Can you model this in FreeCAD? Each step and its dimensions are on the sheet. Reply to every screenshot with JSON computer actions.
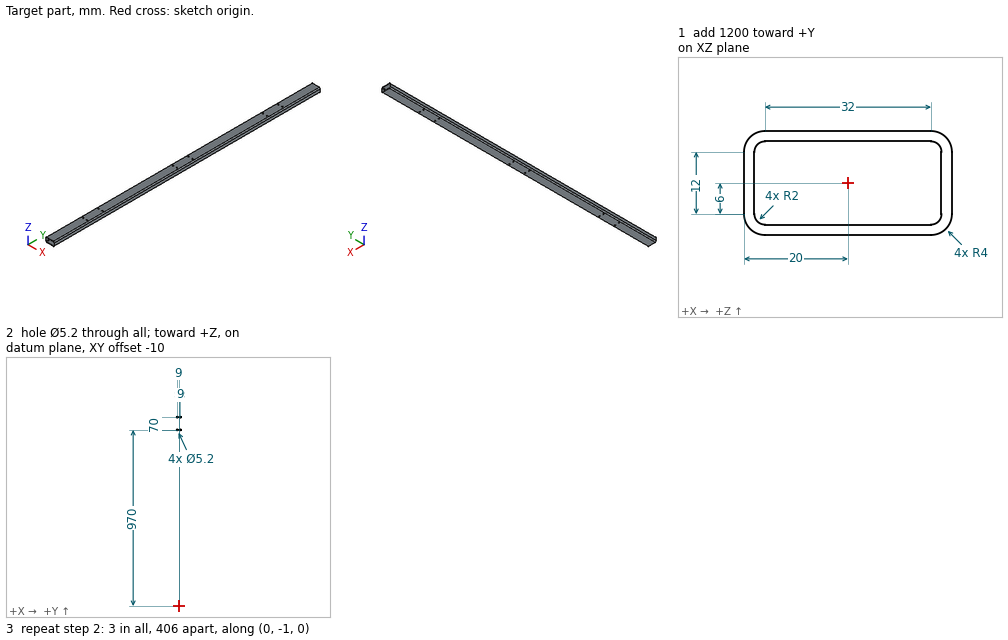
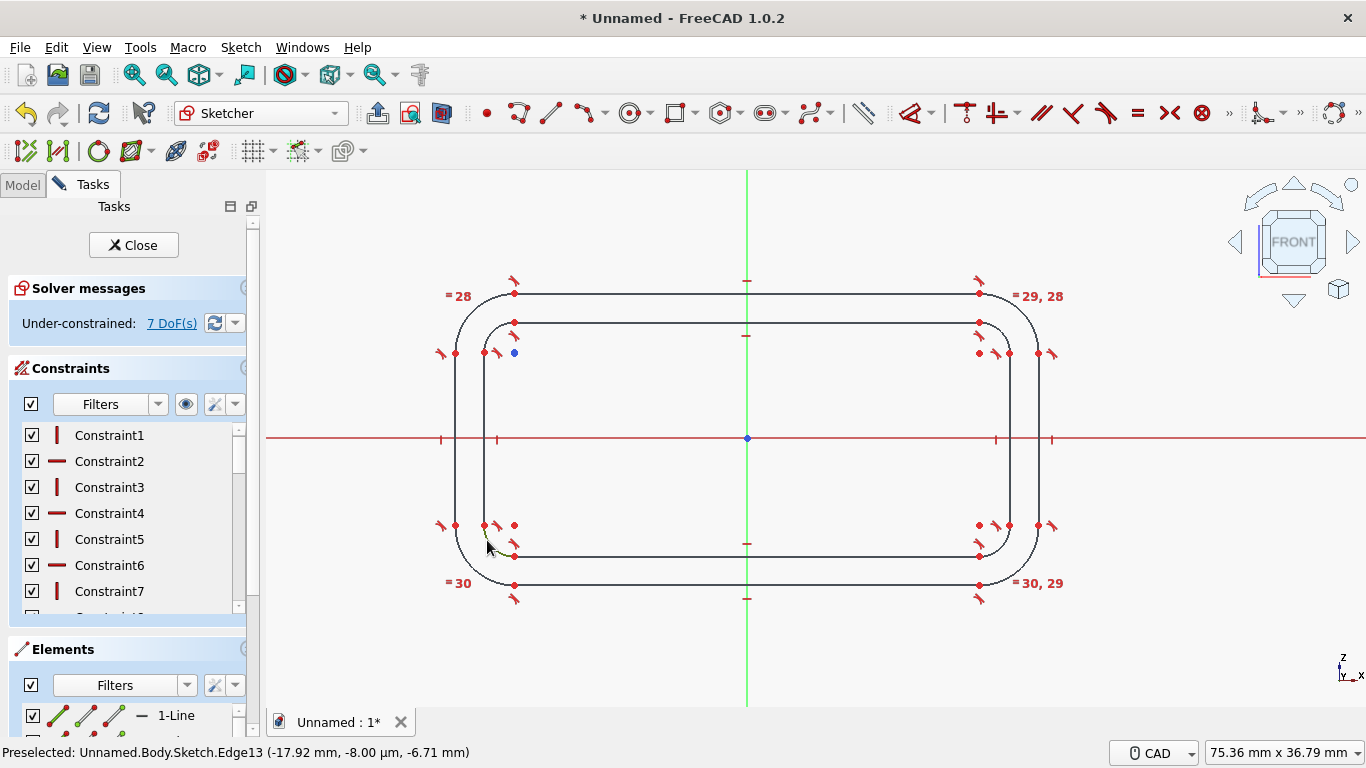
{"action": "left_click", "coordinate": [501, 326]}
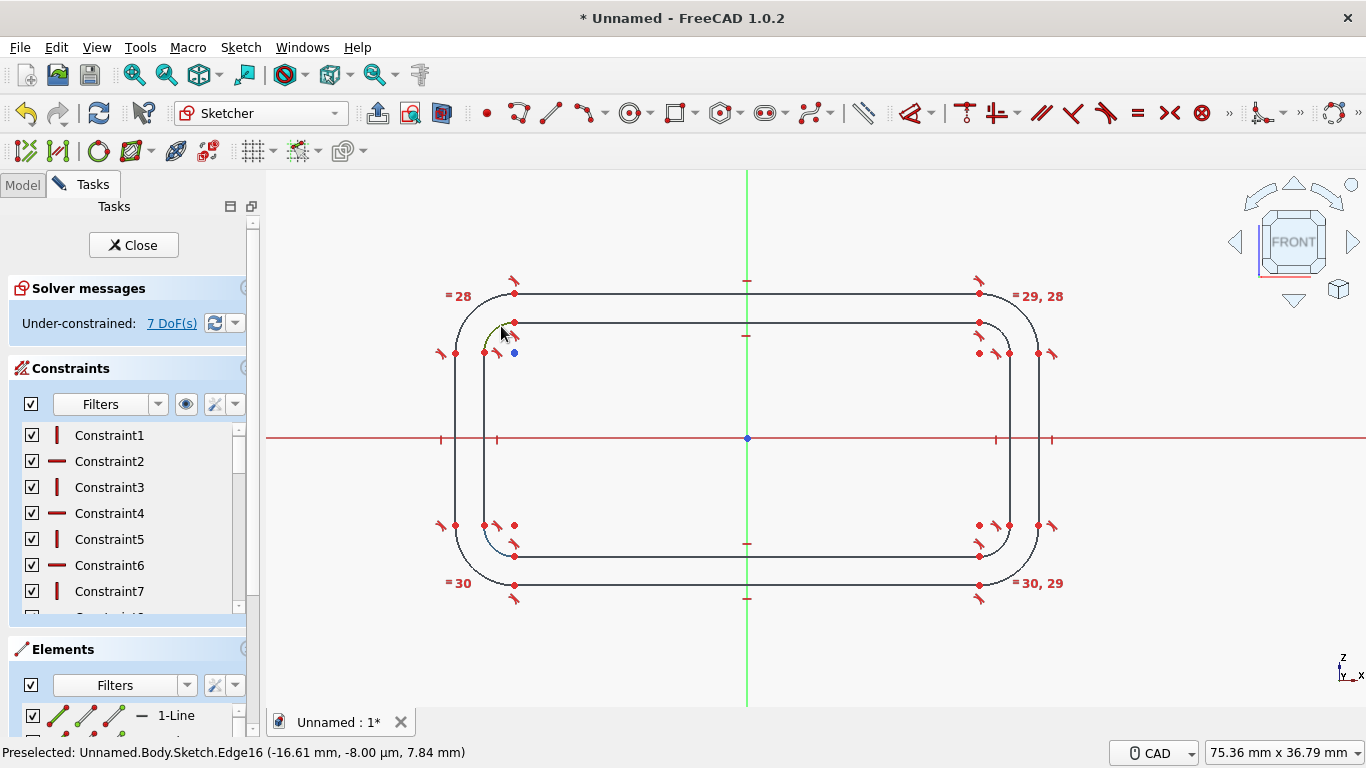
{"action": "left_click", "coordinate": [1138, 114]}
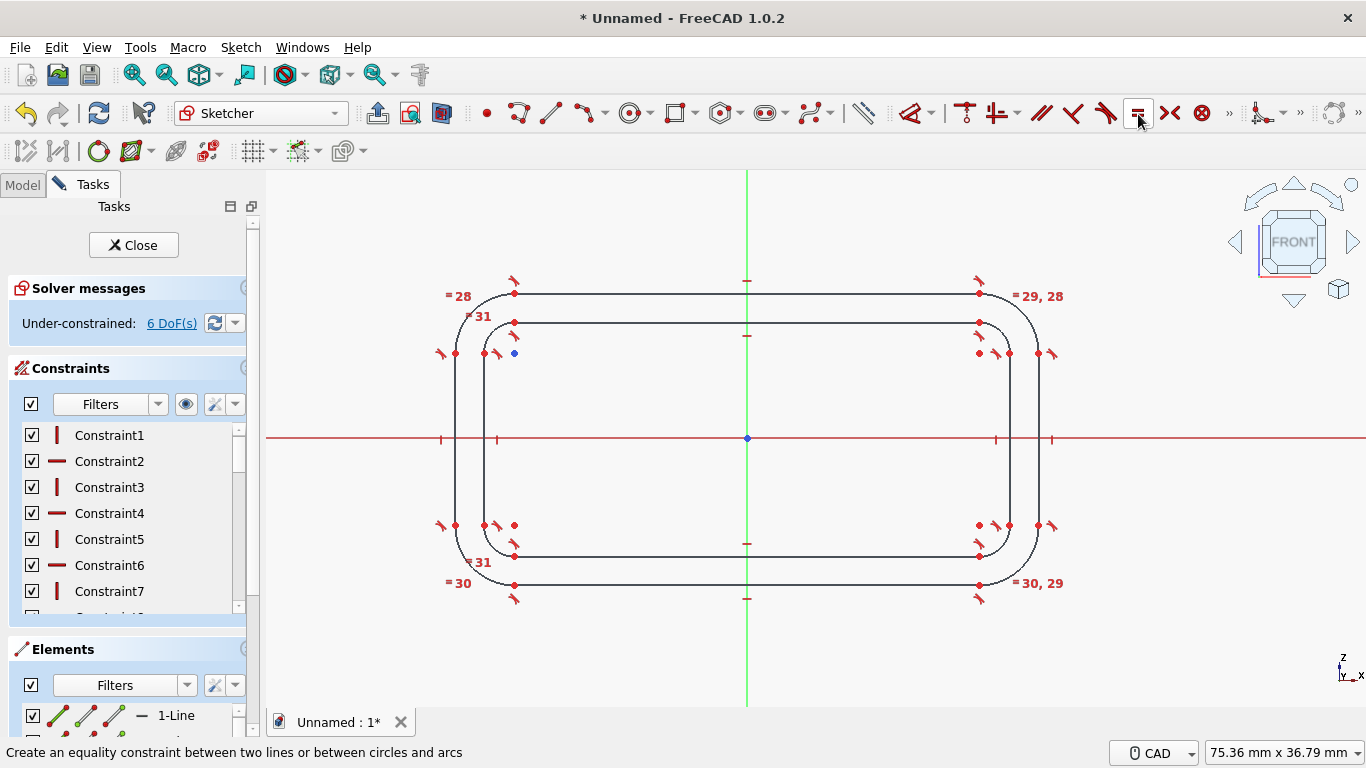
{"action": "left_click", "coordinate": [910, 114]}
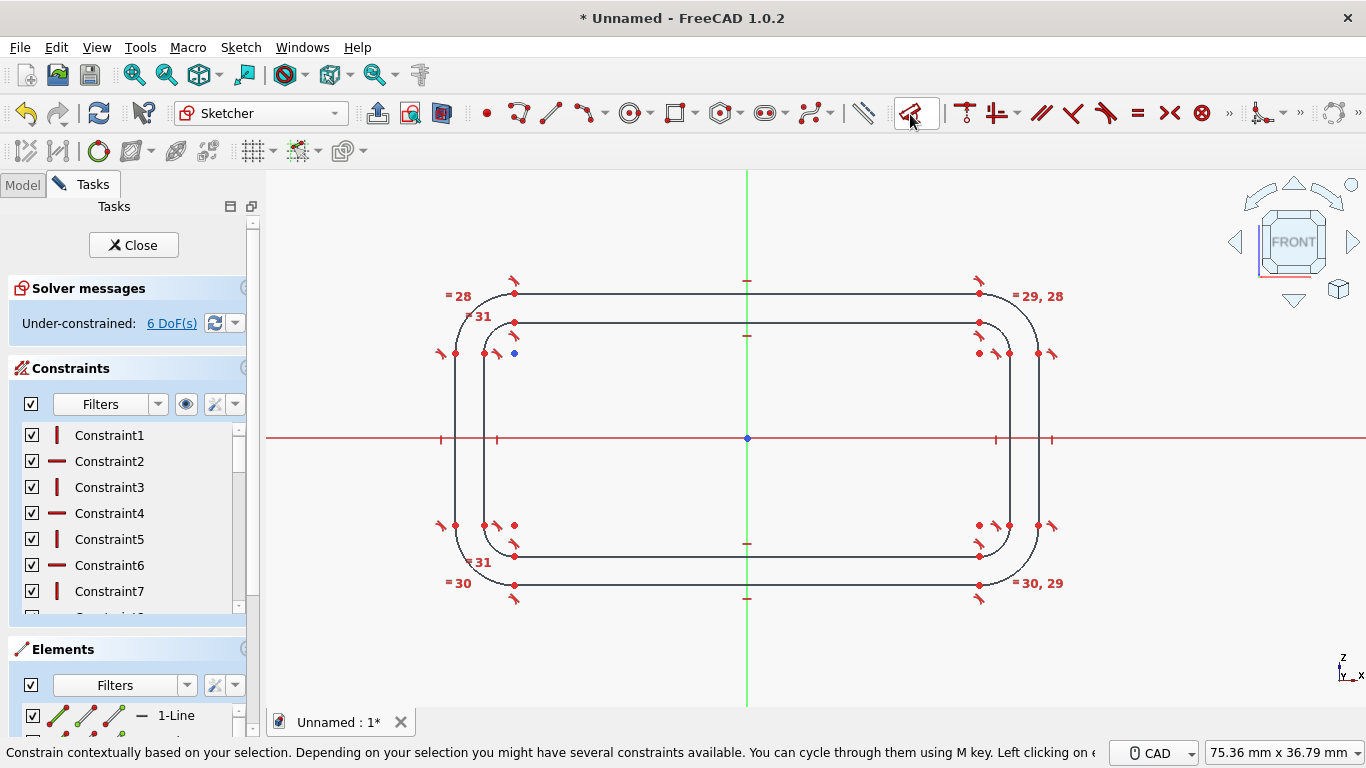
{"action": "left_click", "coordinate": [488, 300]}
{"action": "left_click", "coordinate": [474, 271]}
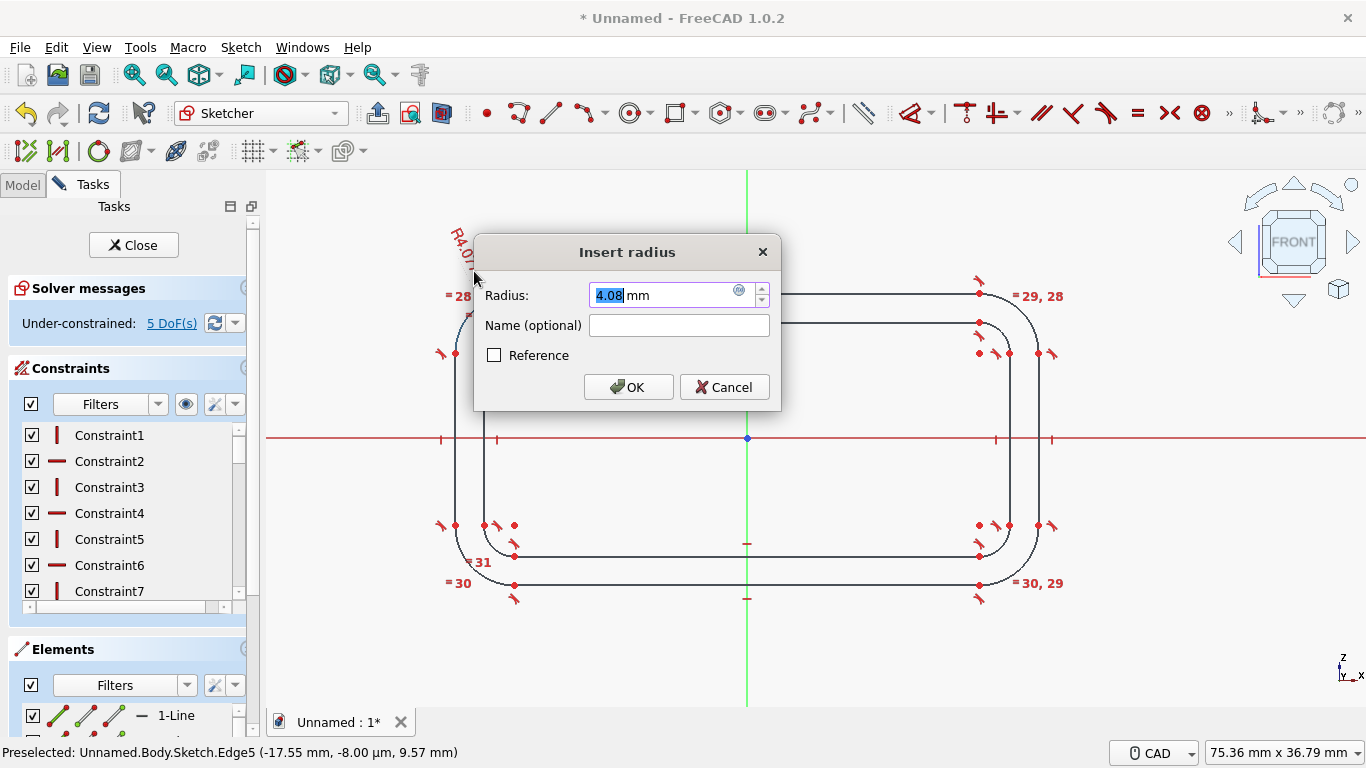
{"action": "type", "text": "4"}
{"action": "key", "text": "Return"}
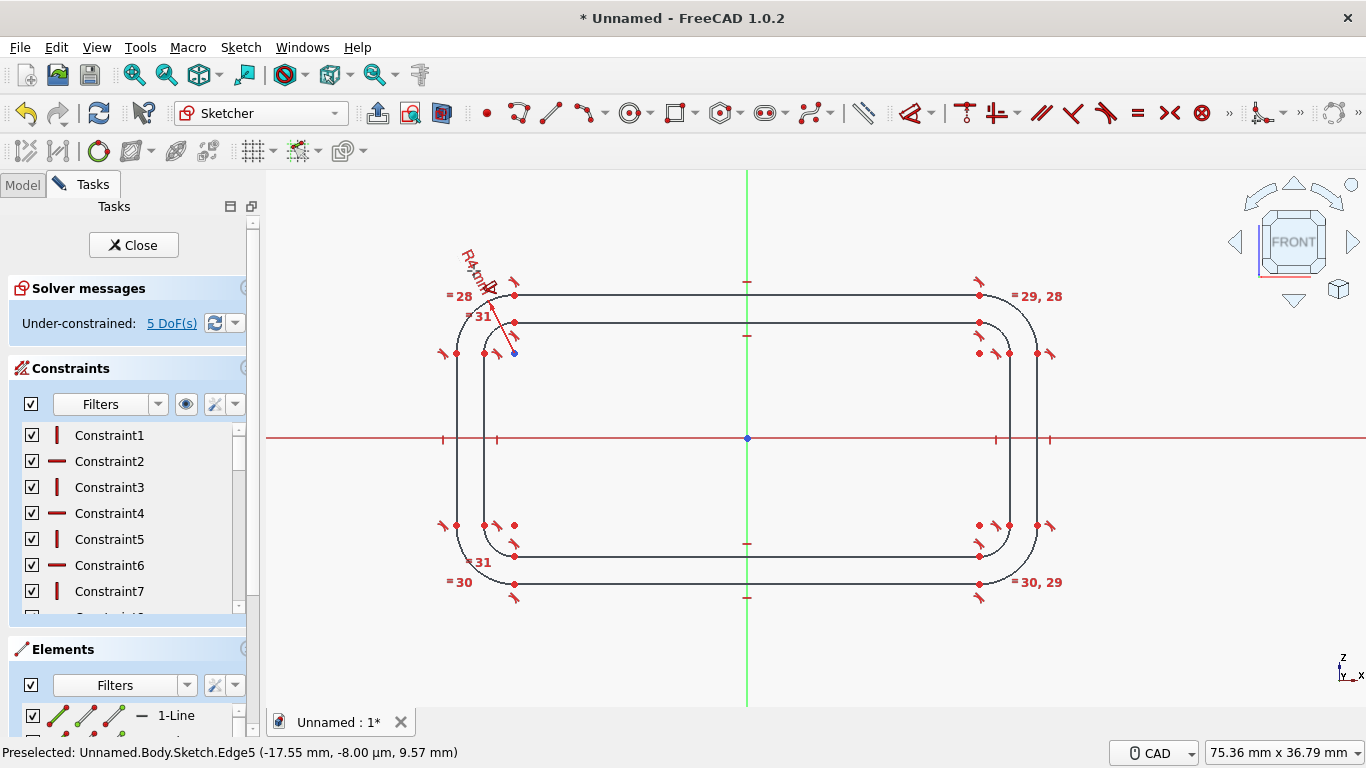
{"action": "scroll", "coordinate": [487, 540], "scroll_direction": "up", "scroll_amount": 2}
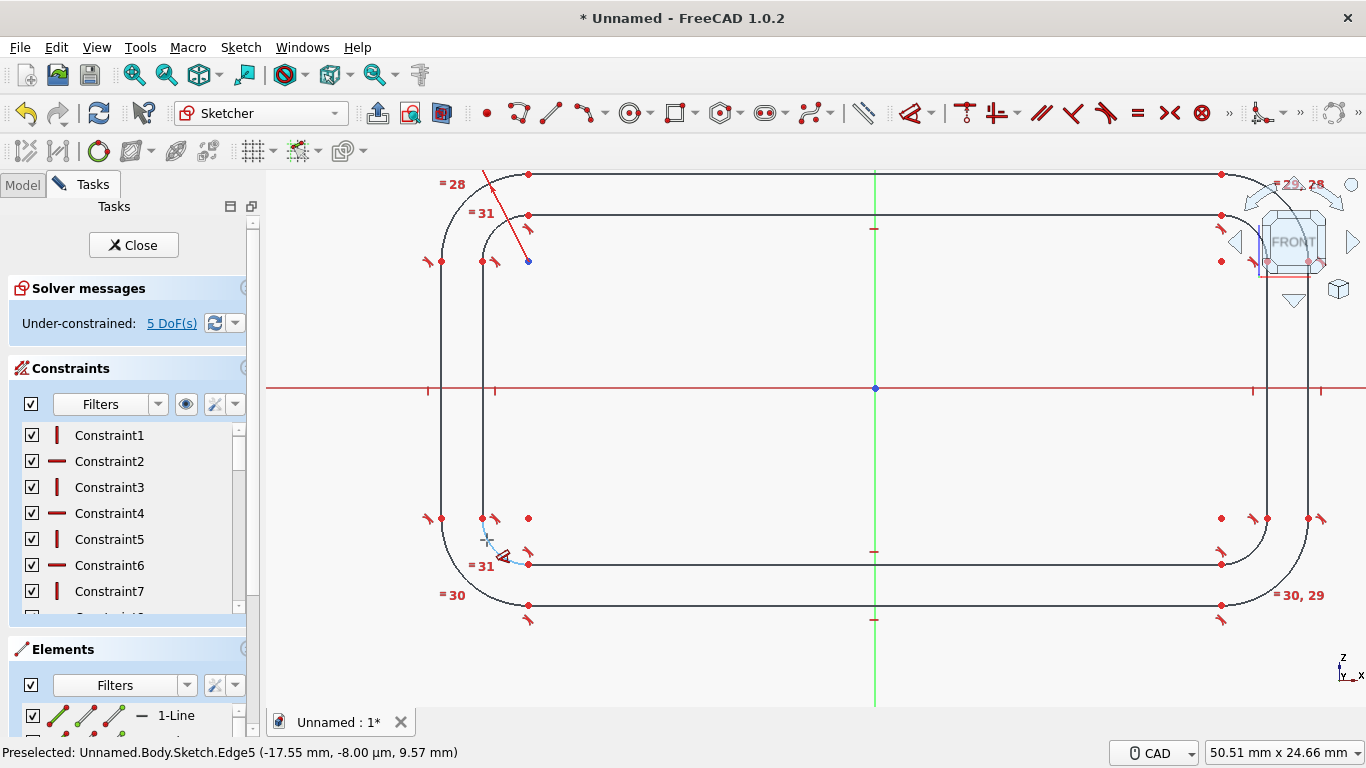
{"action": "left_click", "coordinate": [488, 540]}
{"action": "left_click", "coordinate": [461, 480]}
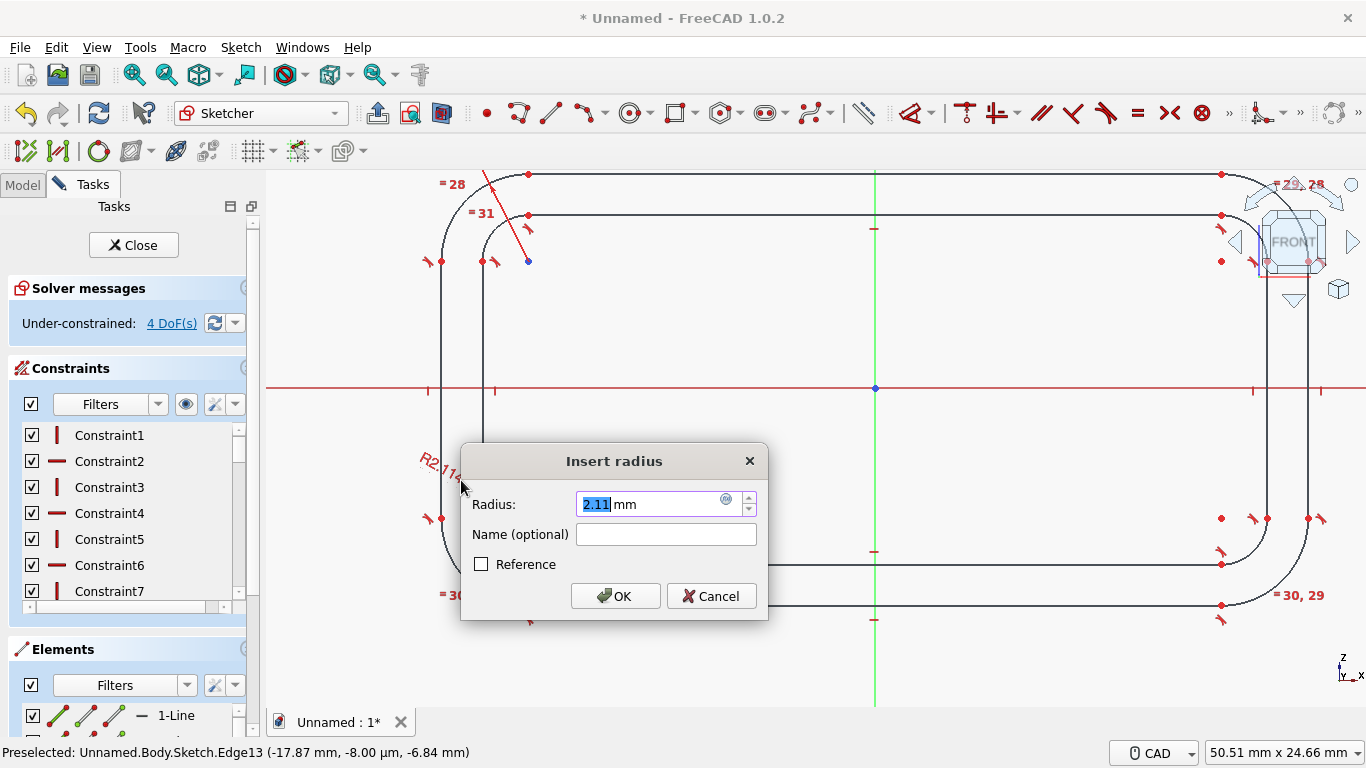
{"action": "type", "text": "2"}
{"action": "key", "text": "Return"}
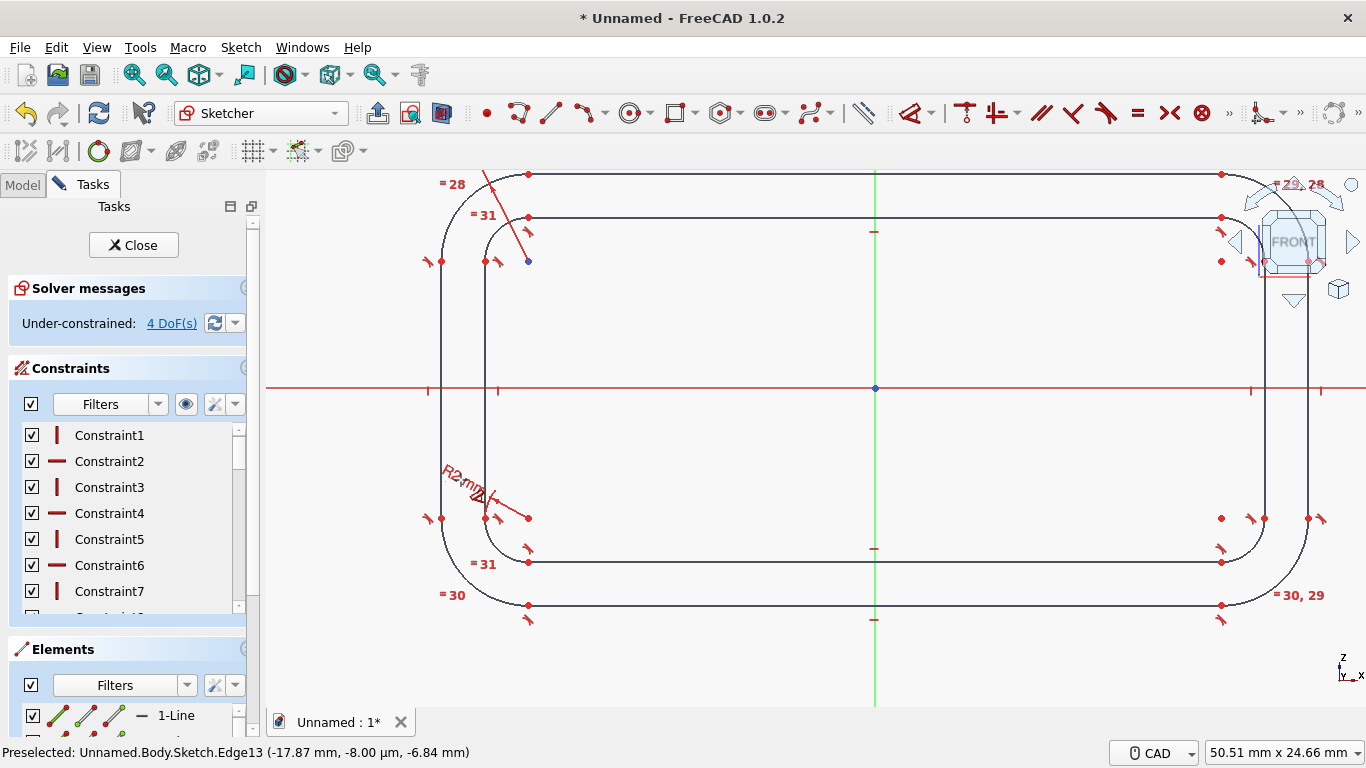
{"action": "left_click", "coordinate": [441, 441]}
{"action": "left_click", "coordinate": [407, 331]}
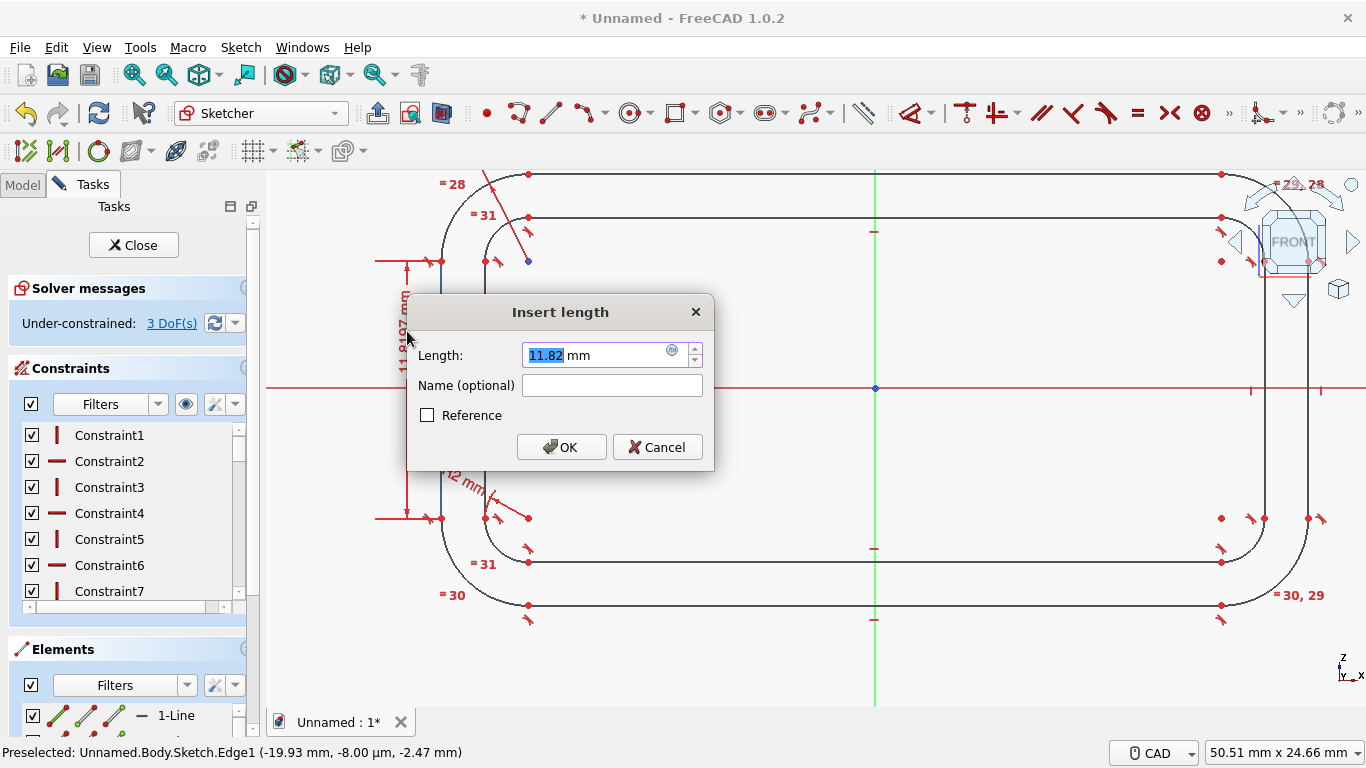
{"action": "type", "text": "12"}
{"action": "key", "text": "Return"}